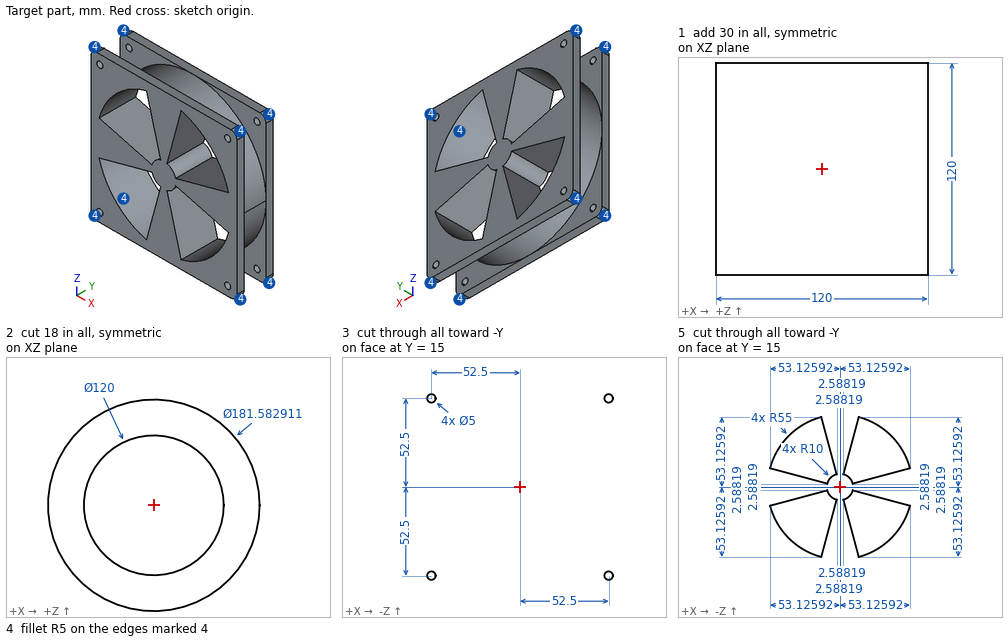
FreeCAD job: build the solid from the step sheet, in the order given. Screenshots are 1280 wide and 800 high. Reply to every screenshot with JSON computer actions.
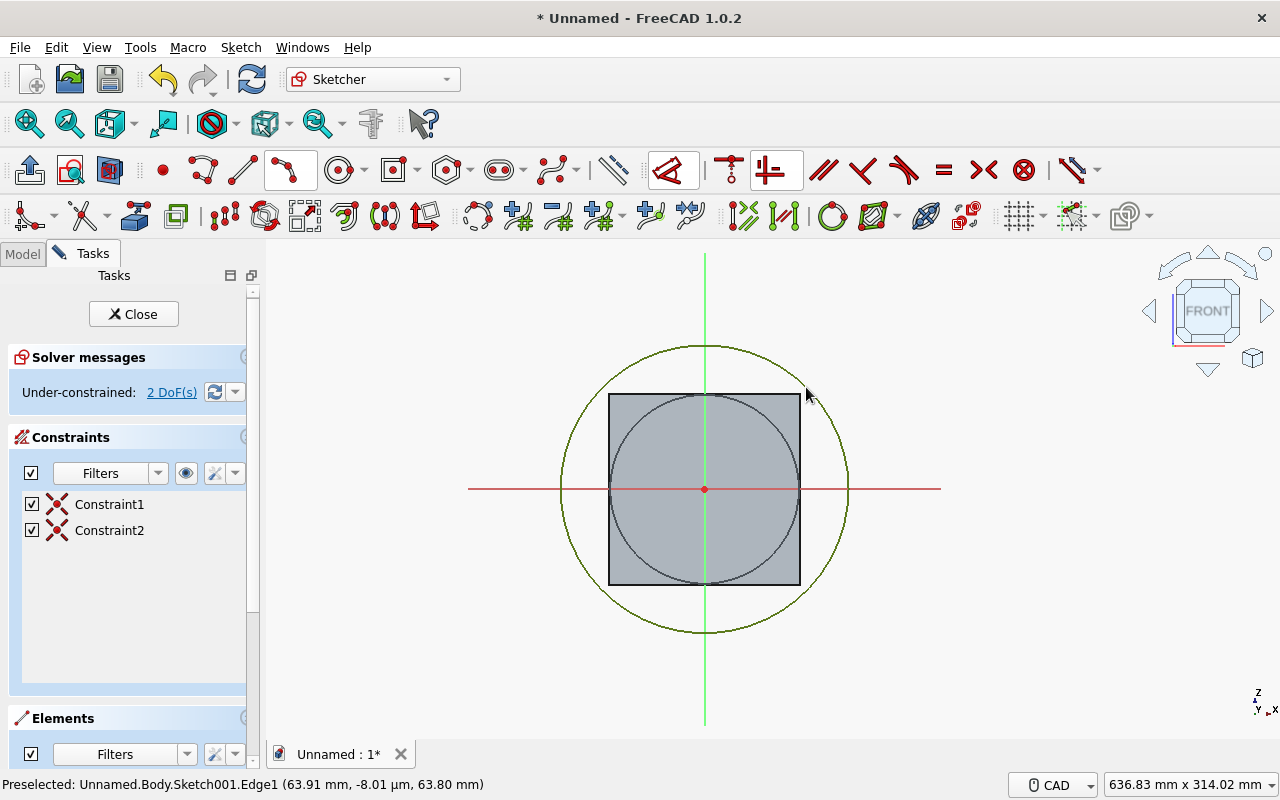
{"action": "left_click", "coordinate": [694, 170]}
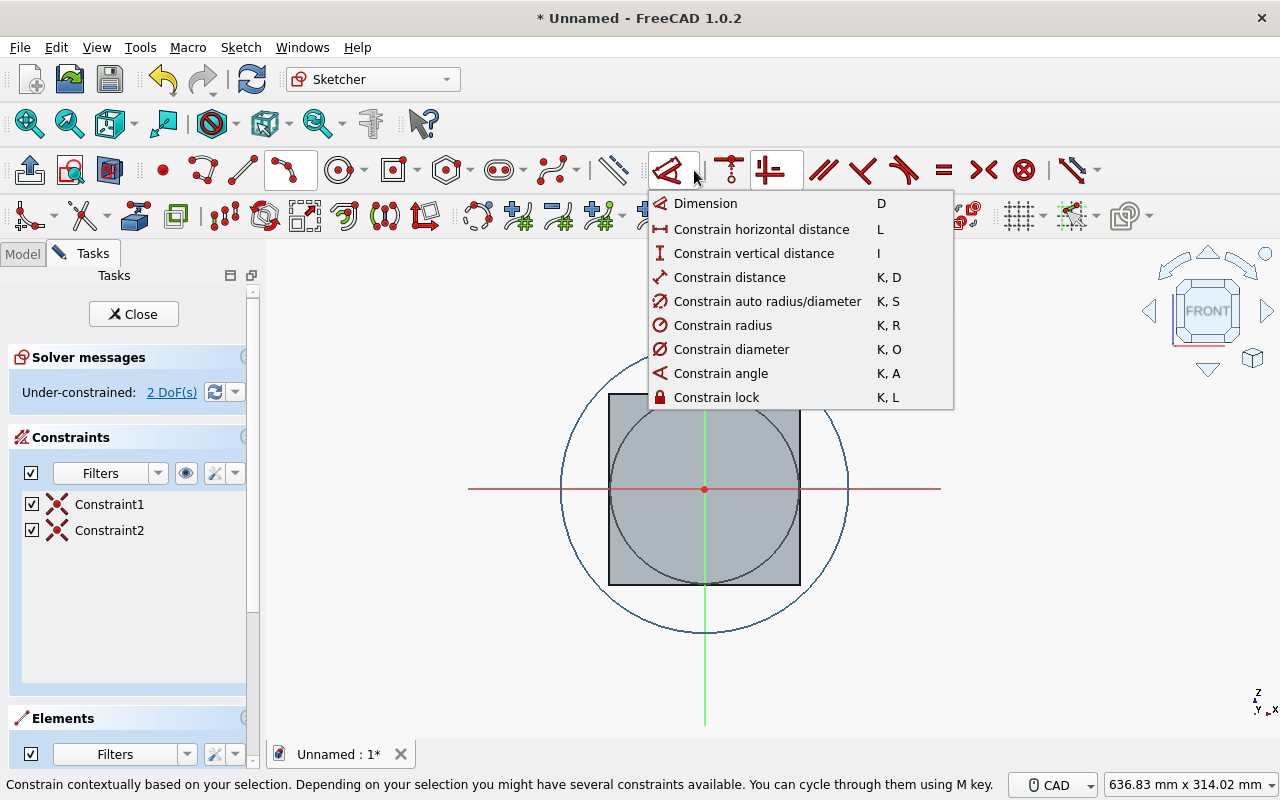
{"action": "left_click", "coordinate": [801, 349]}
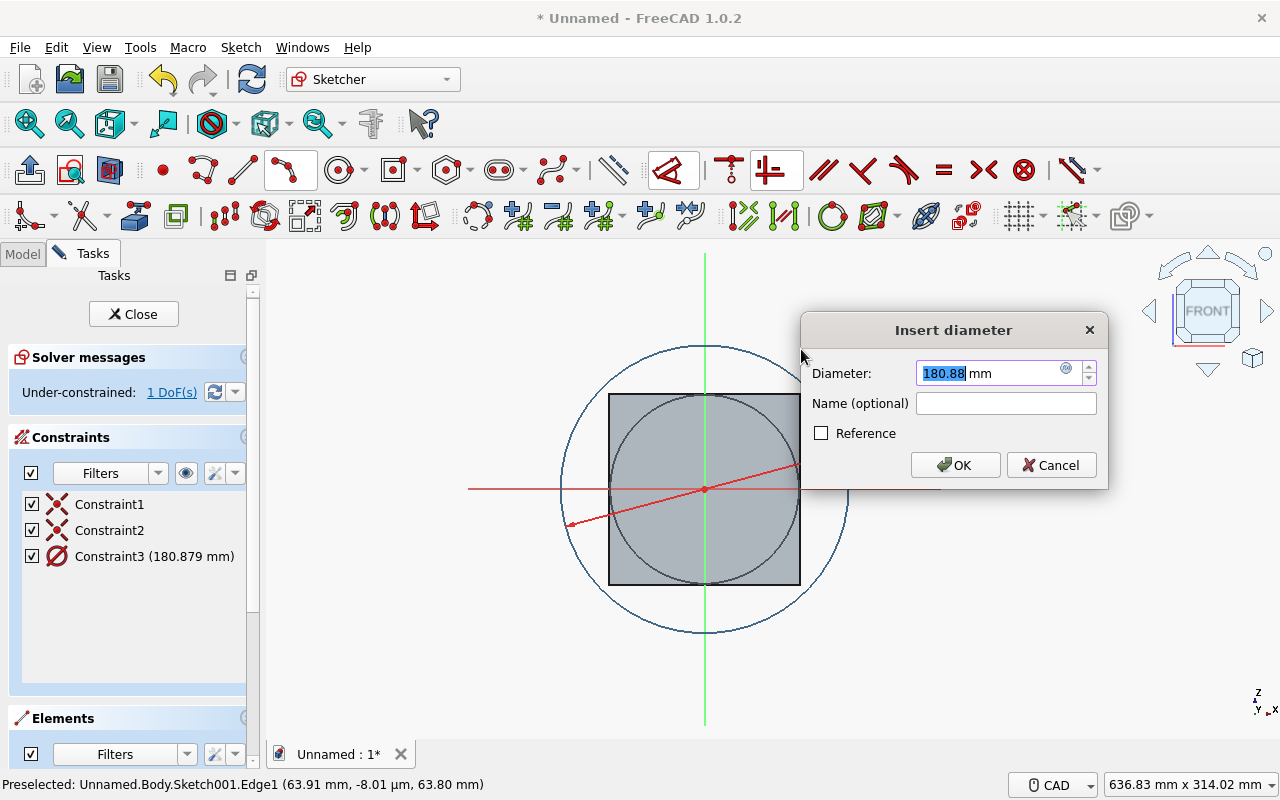
{"action": "type", "text": "181.582911"}
{"action": "key", "text": "Return"}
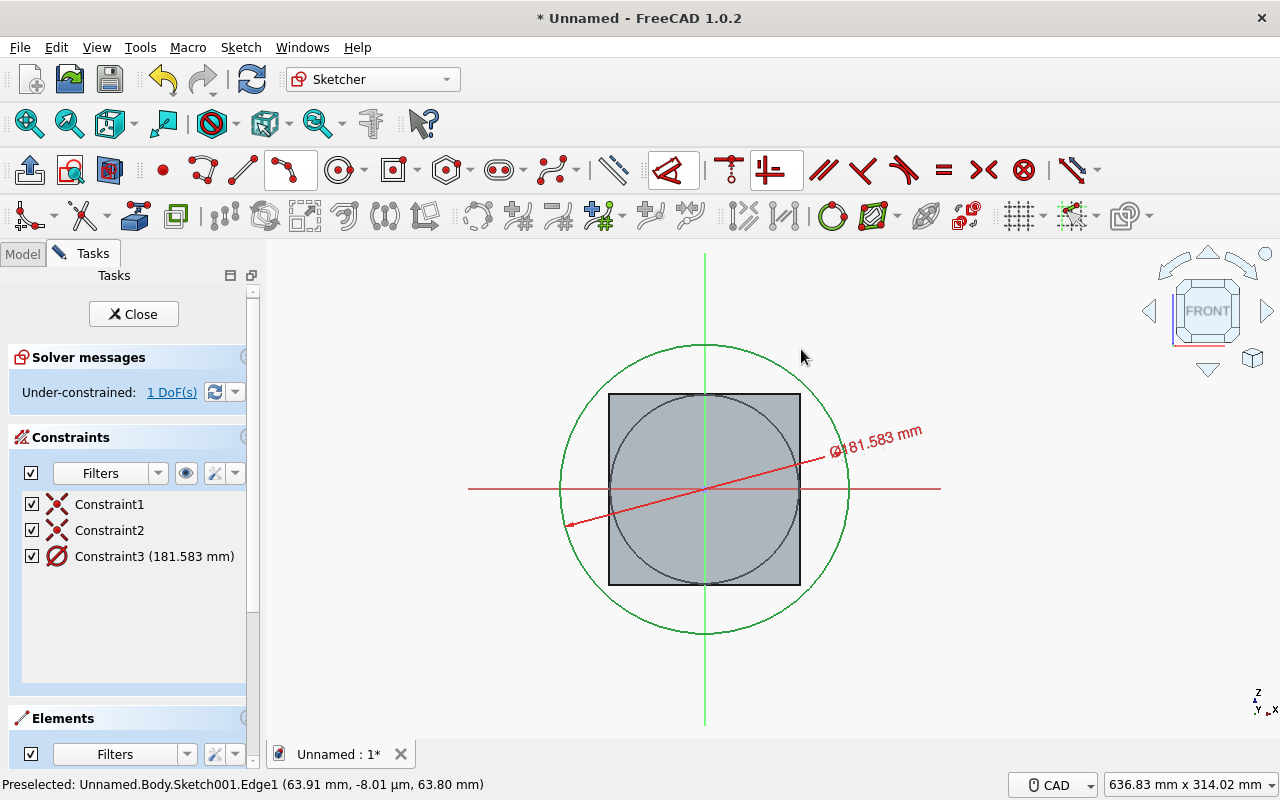
{"action": "left_click", "coordinate": [771, 422]}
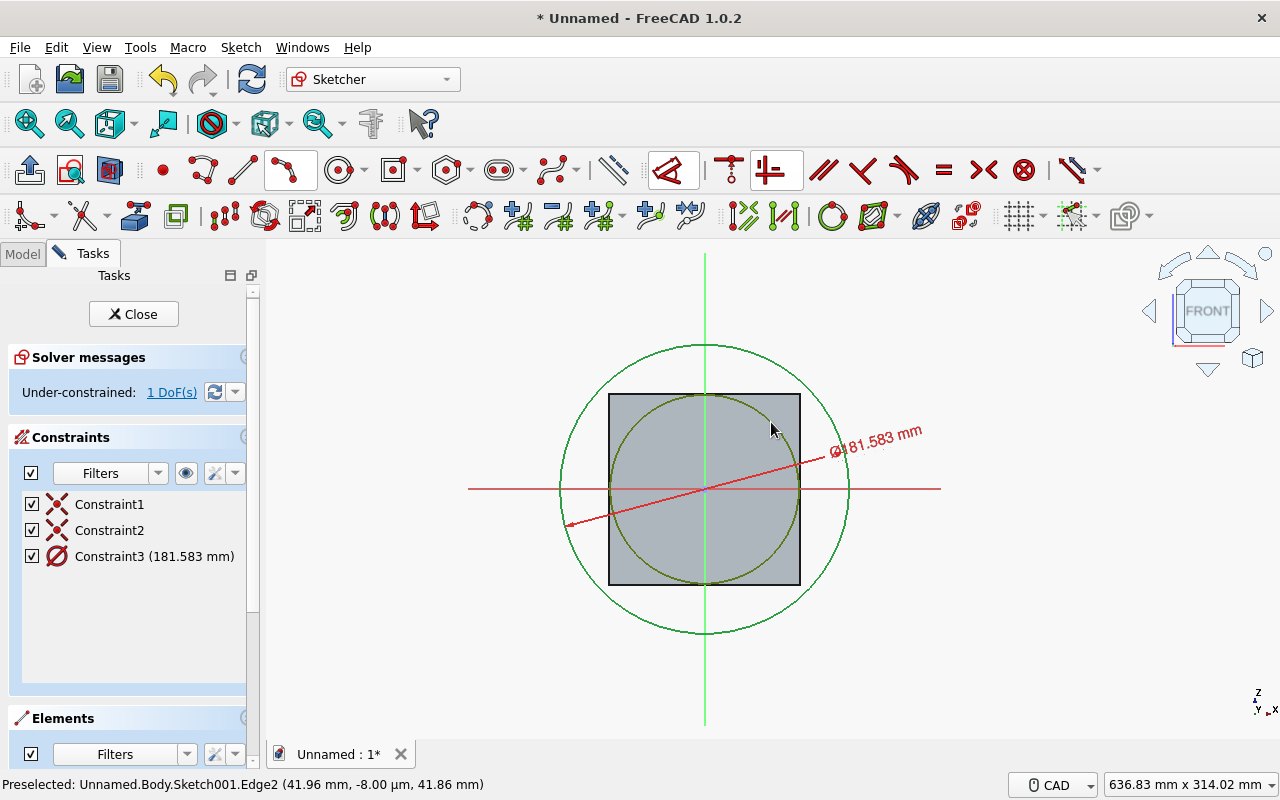
{"action": "left_click", "coordinate": [694, 170]}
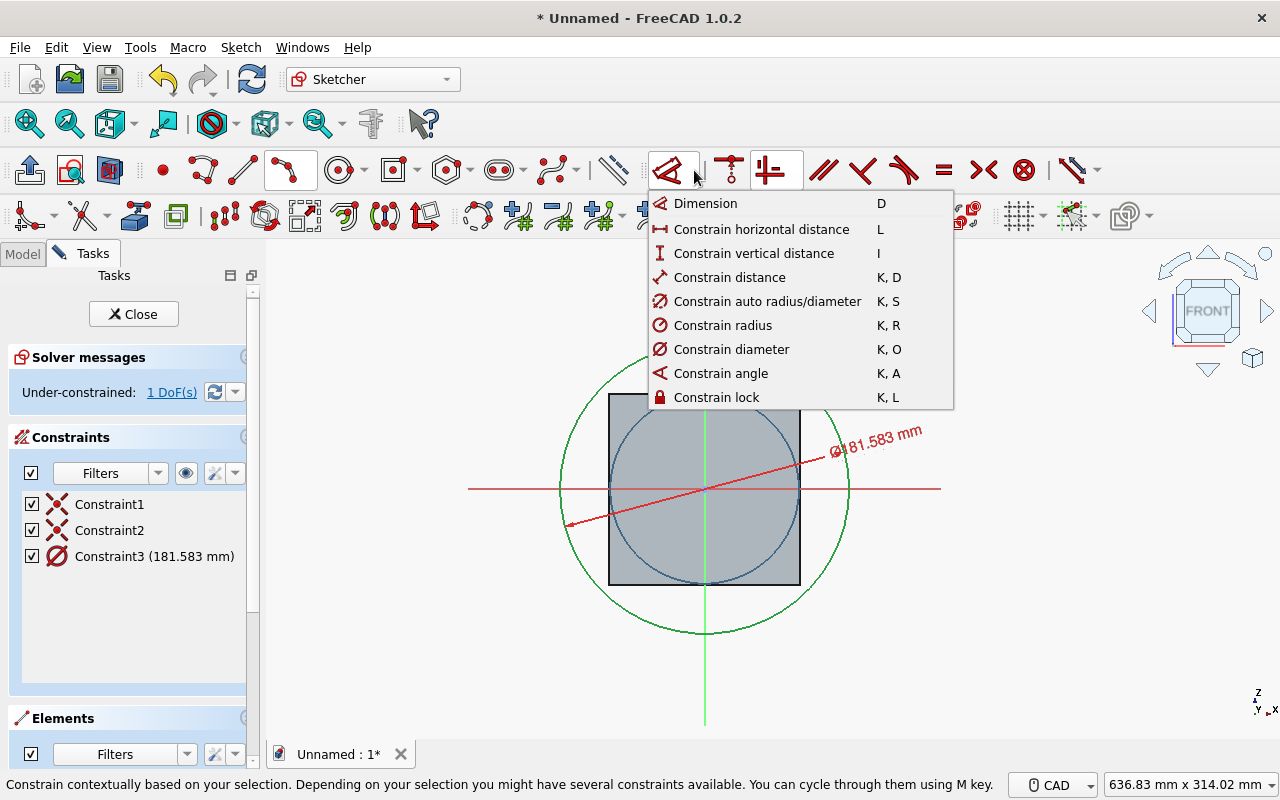
{"action": "left_click", "coordinate": [801, 349]}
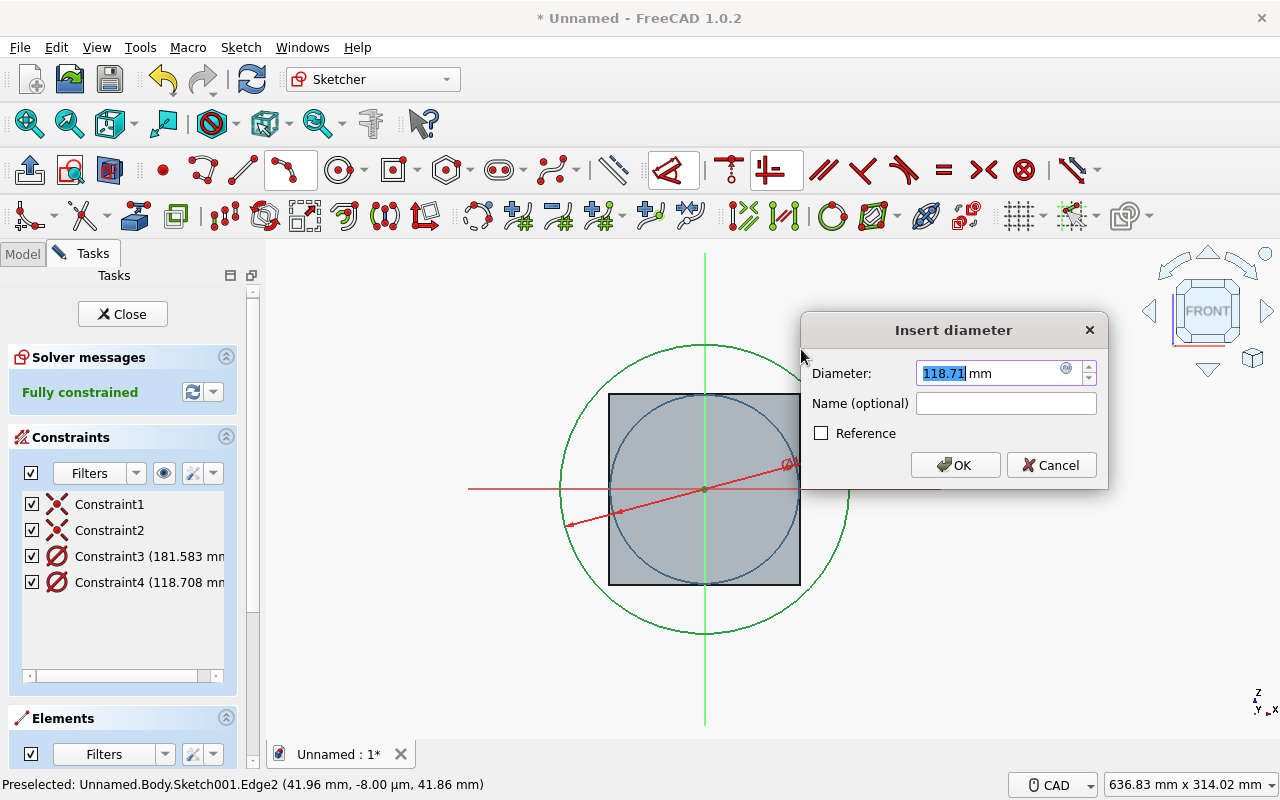
{"action": "type", "text": "120"}
{"action": "key", "text": "Return"}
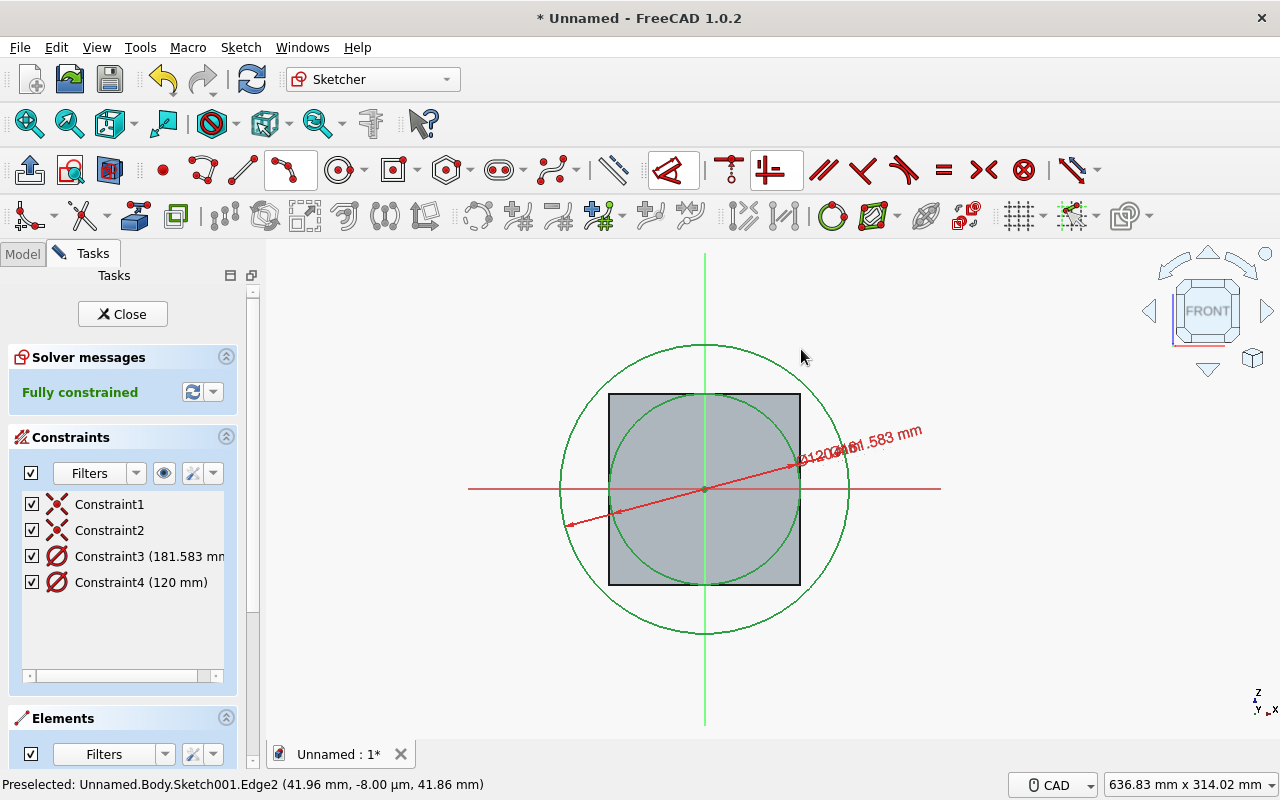
{"action": "left_click", "coordinate": [123, 314]}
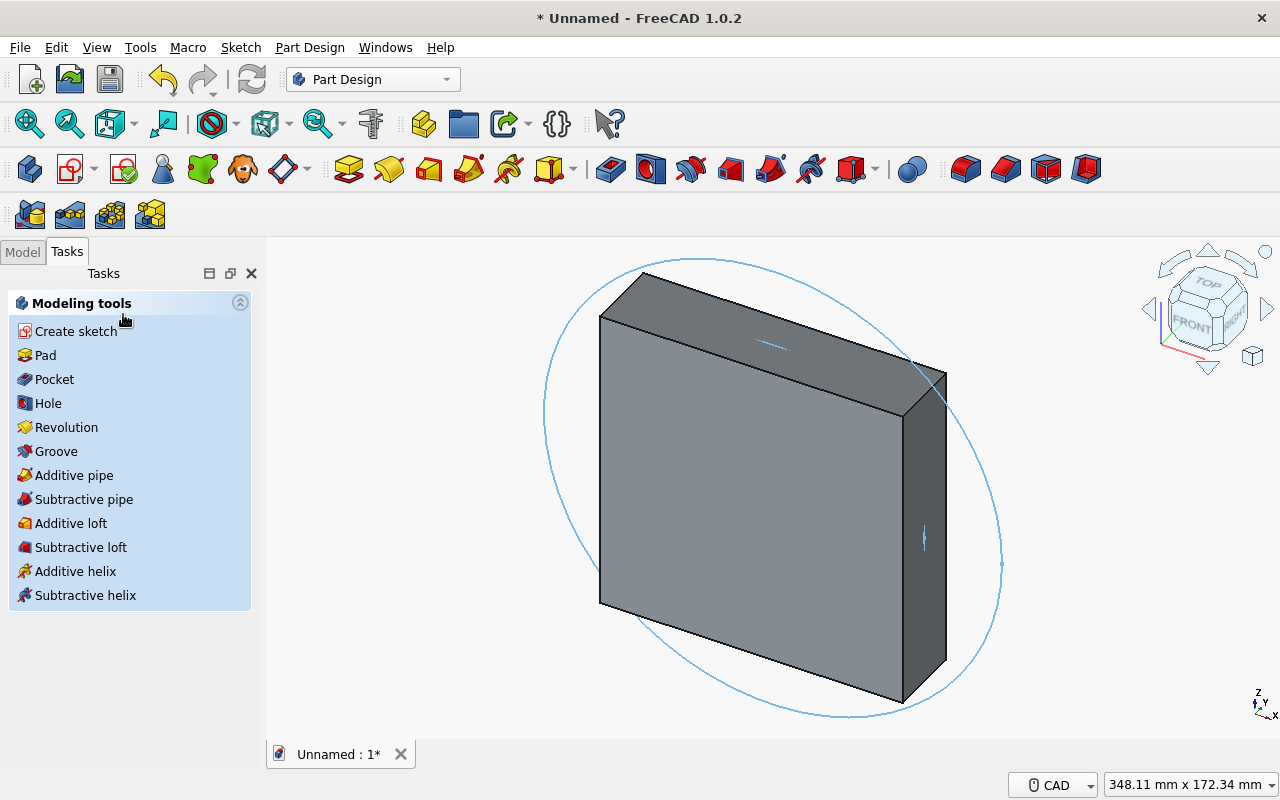
{"action": "left_click", "coordinate": [612, 170]}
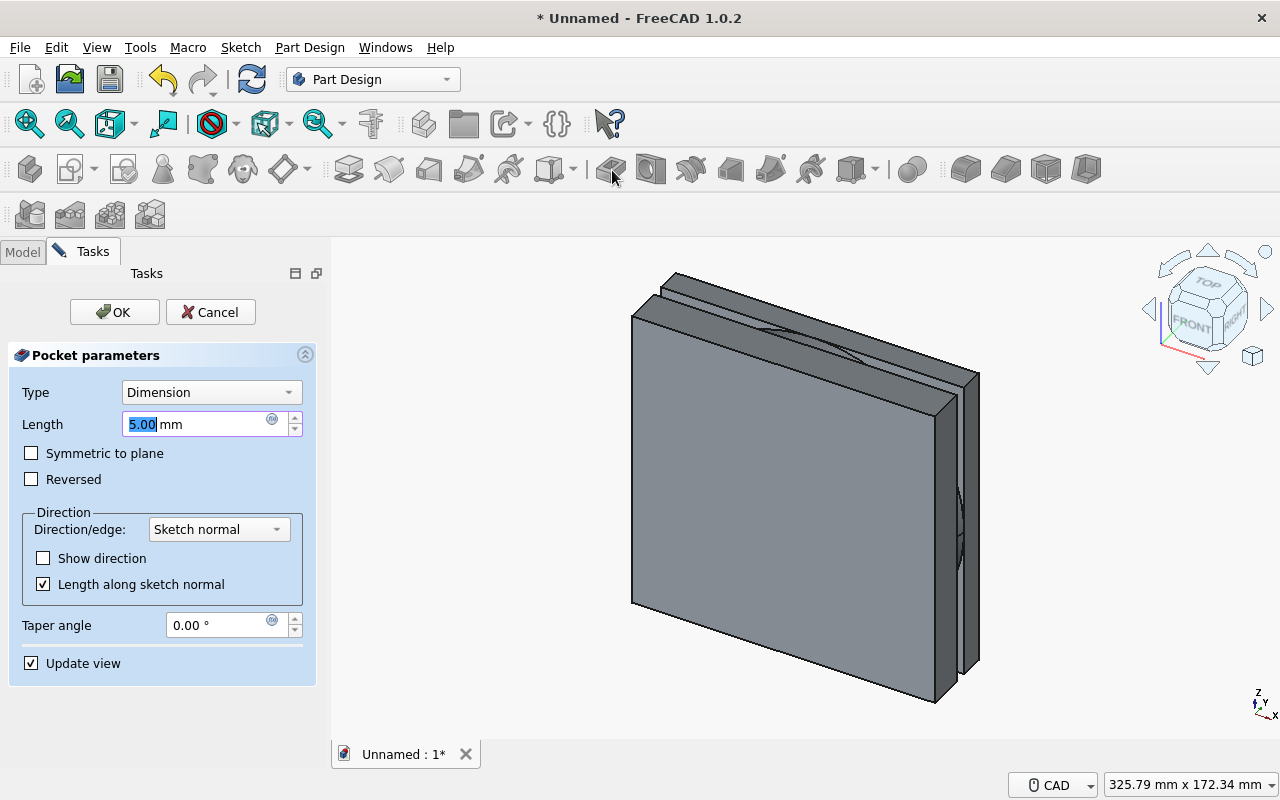
{"action": "type", "text": "18"}
{"action": "key", "text": "Tab"}